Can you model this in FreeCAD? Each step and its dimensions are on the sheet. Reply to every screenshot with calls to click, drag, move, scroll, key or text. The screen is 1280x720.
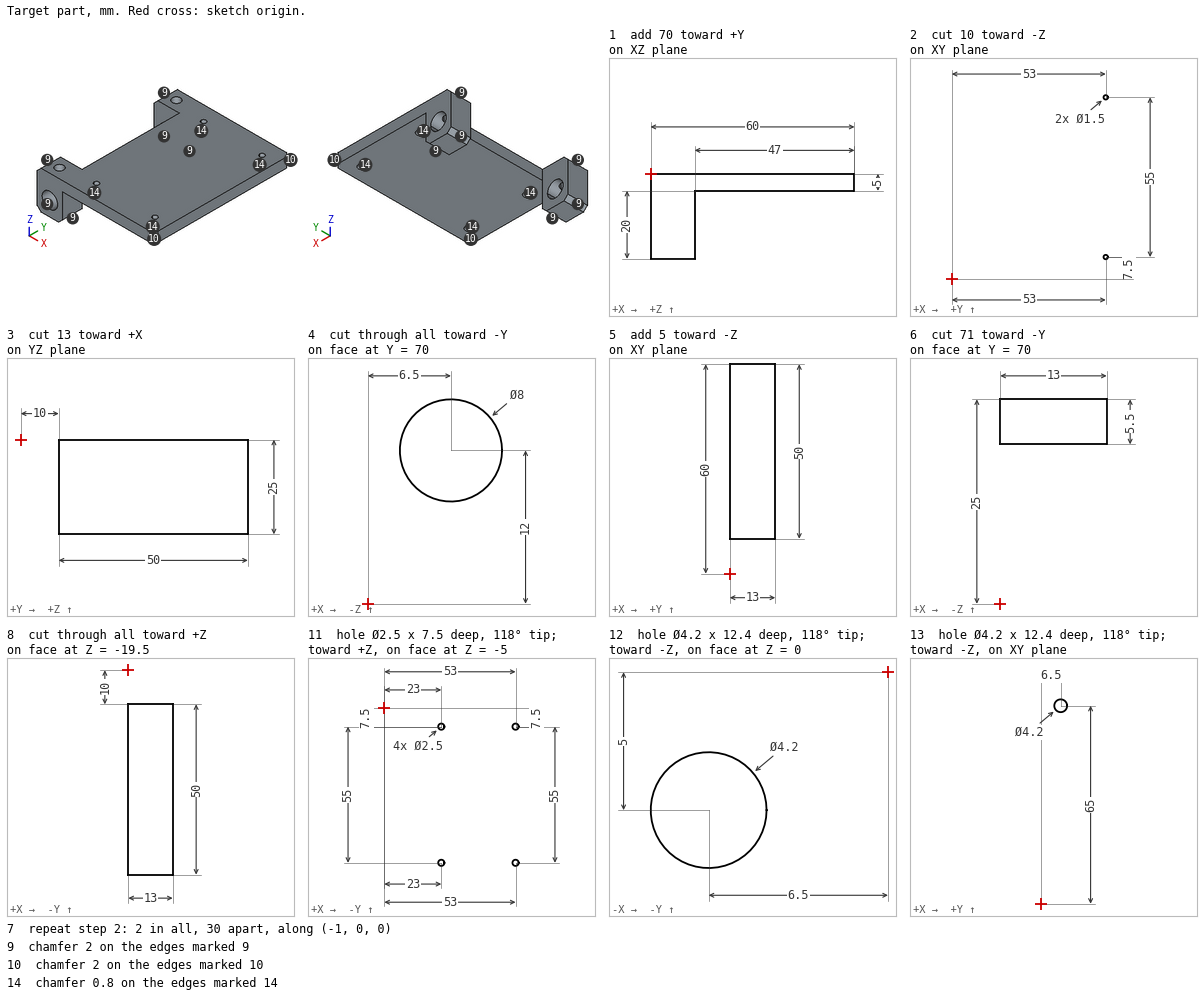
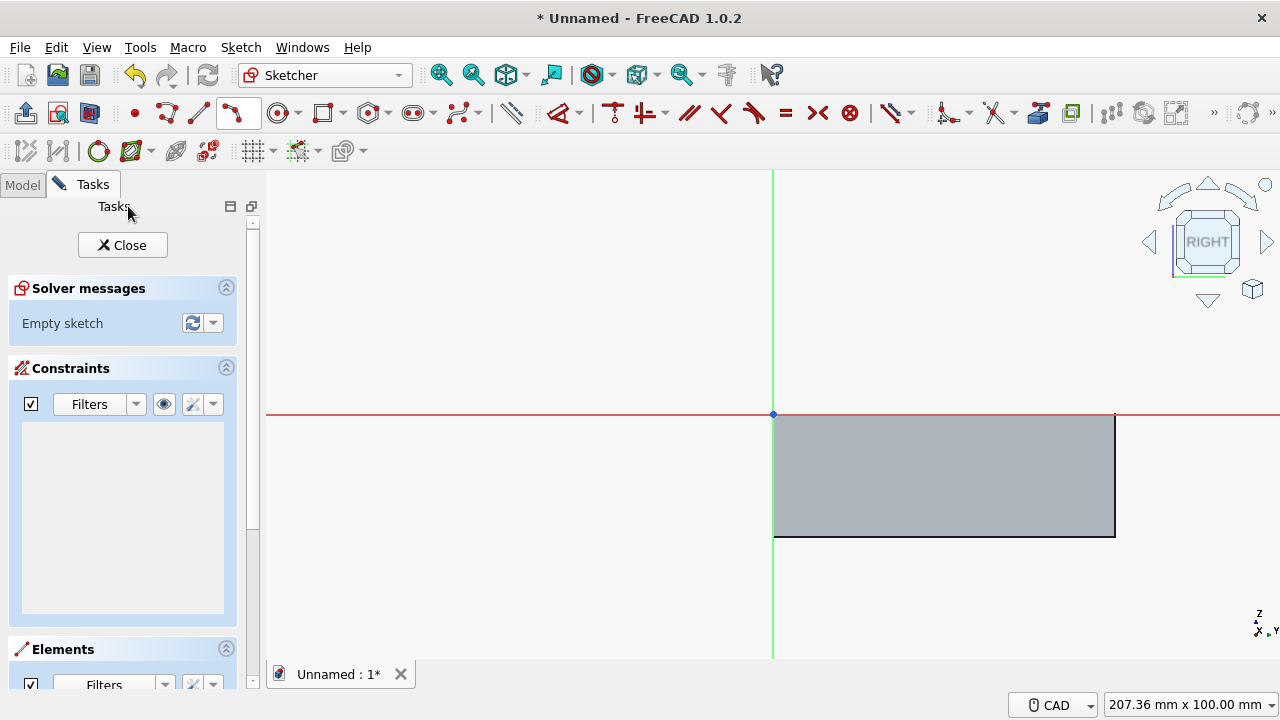
scroll(1115, 550, up, 3)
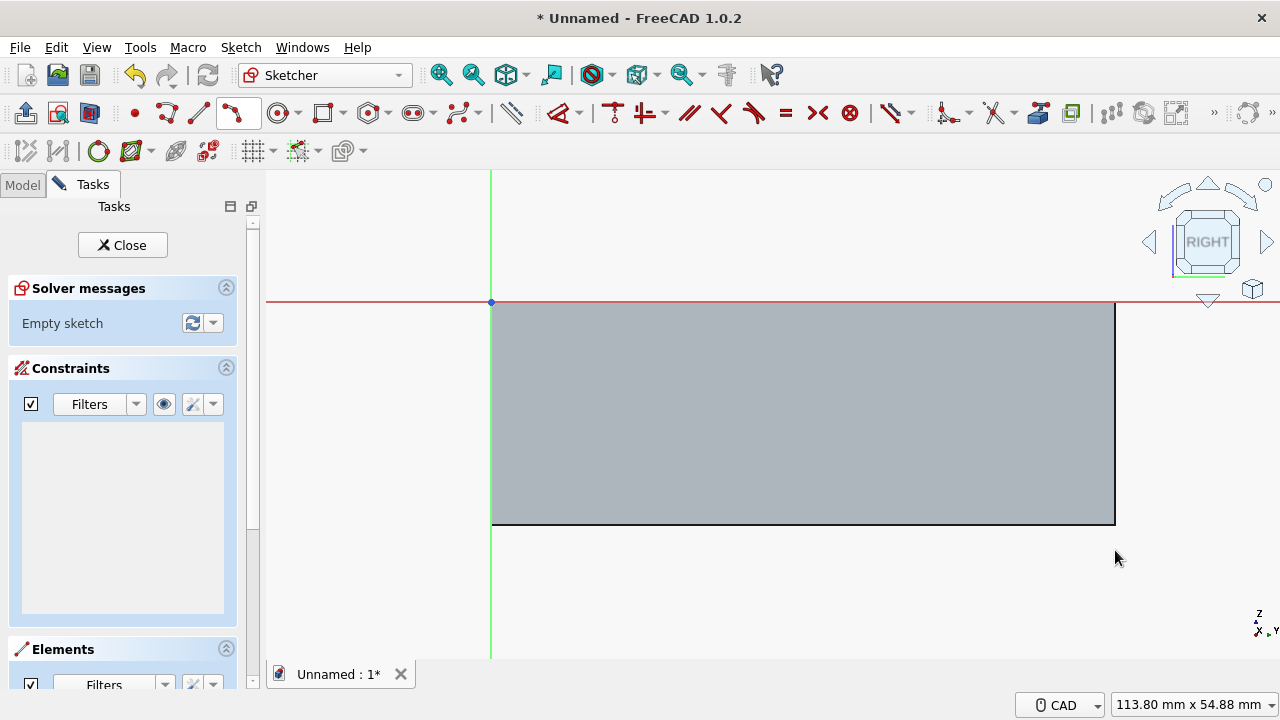
key(g)
key(r)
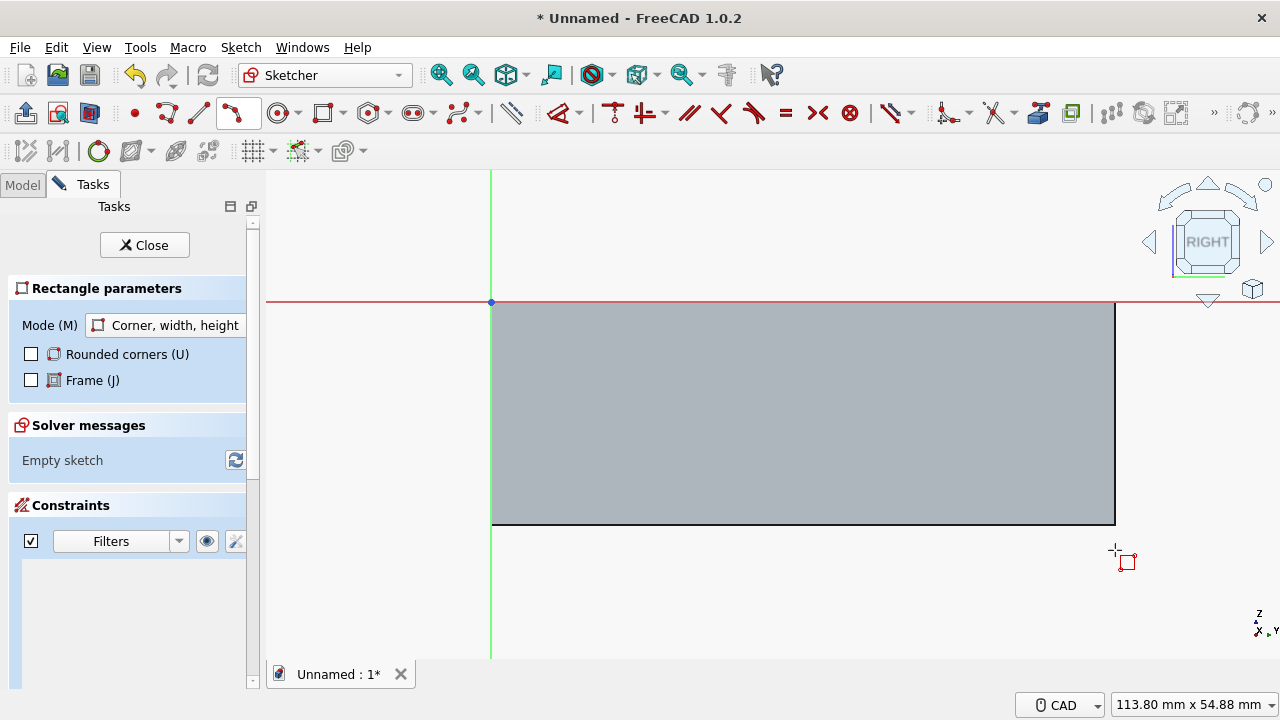
click(580, 302)
move(1026, 525)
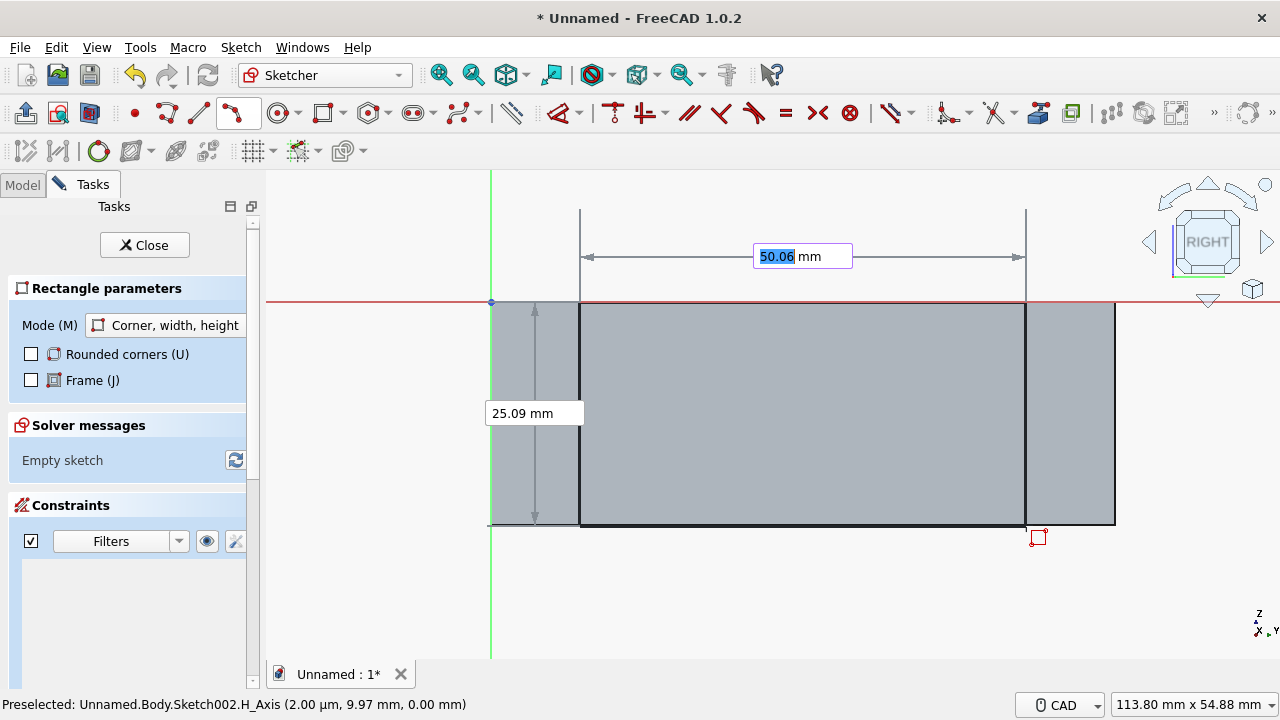
text(50)
key(Tab)
text(25)
key(Return)
key(Escape)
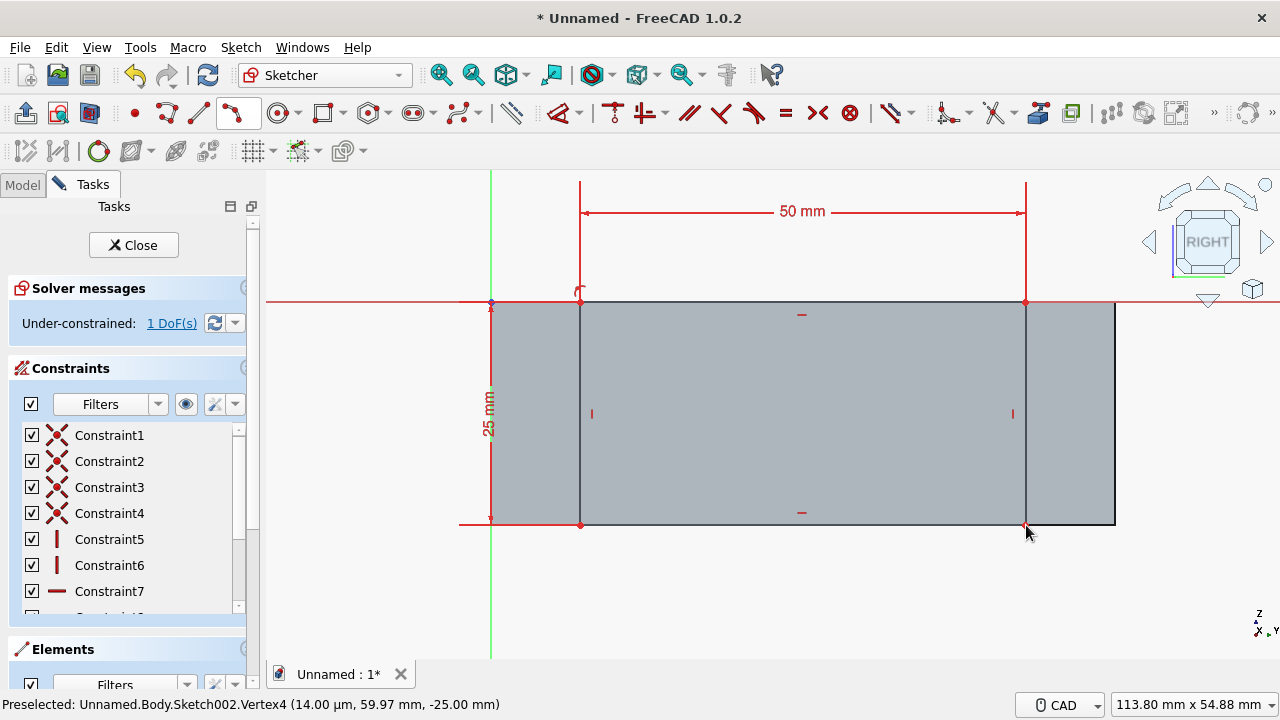
key(d)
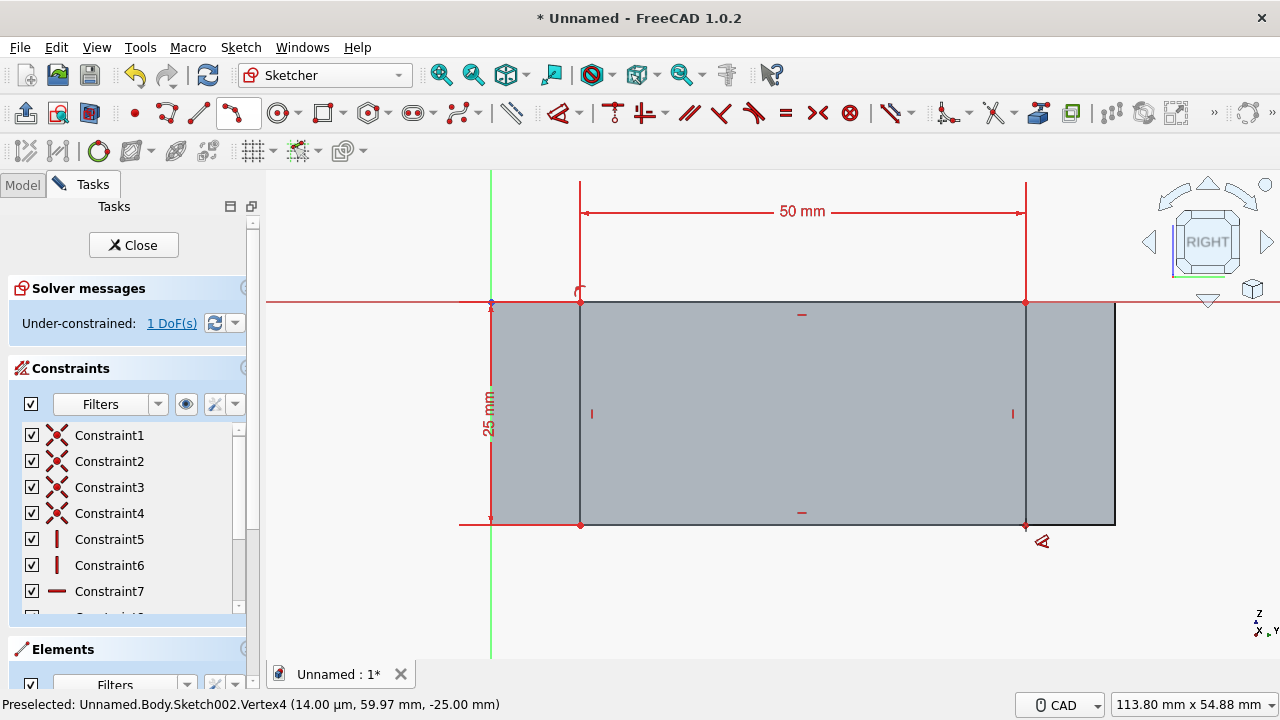
click(580, 302)
click(536, 268)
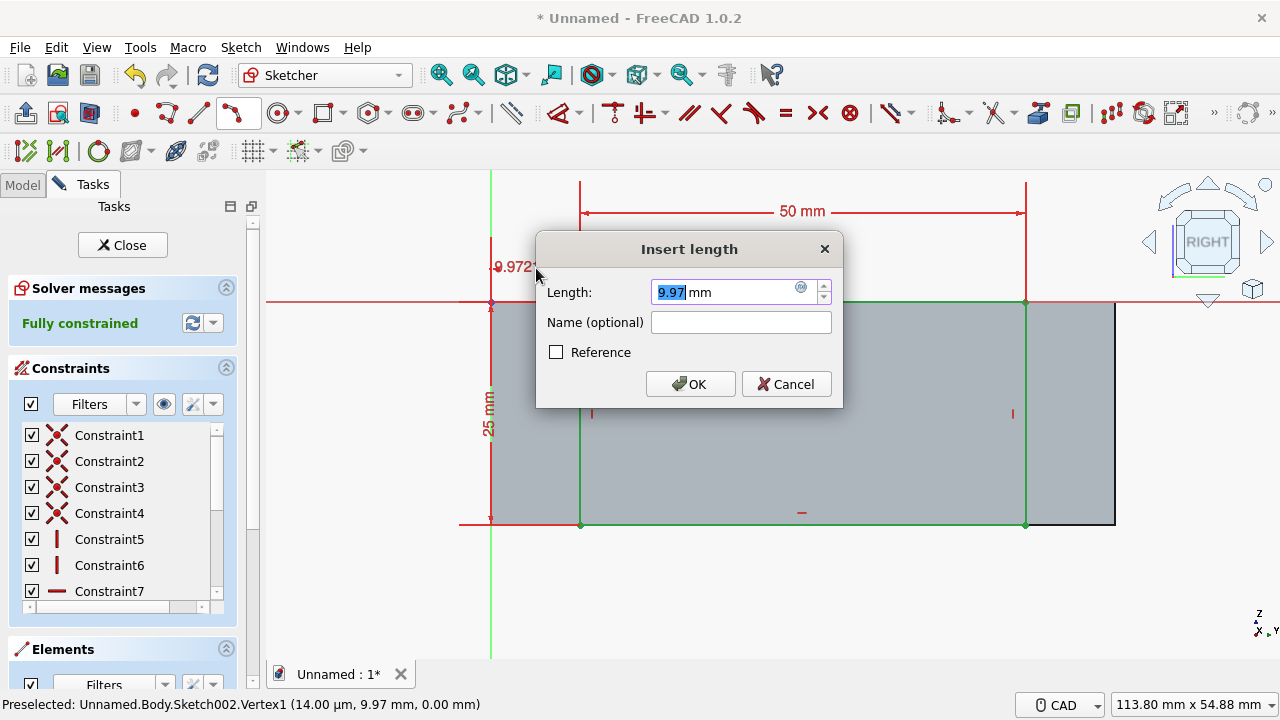
text(10)
key(Return)
key(Escape)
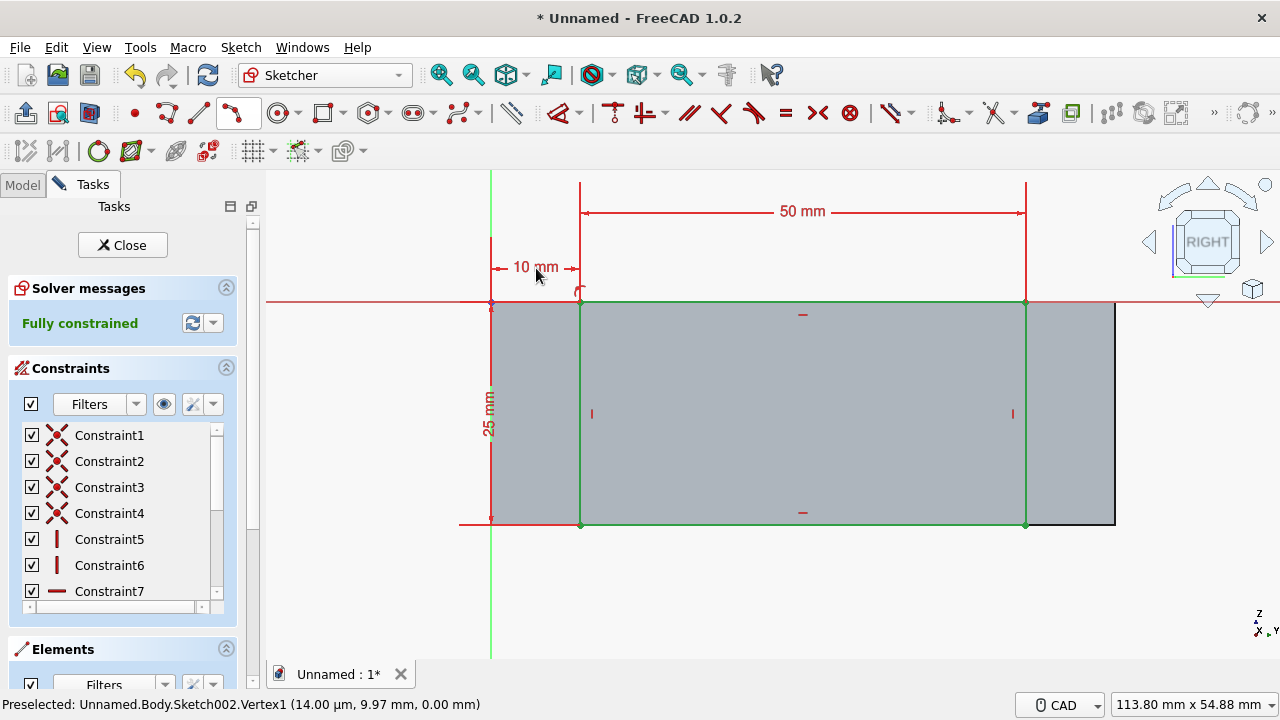
click(123, 245)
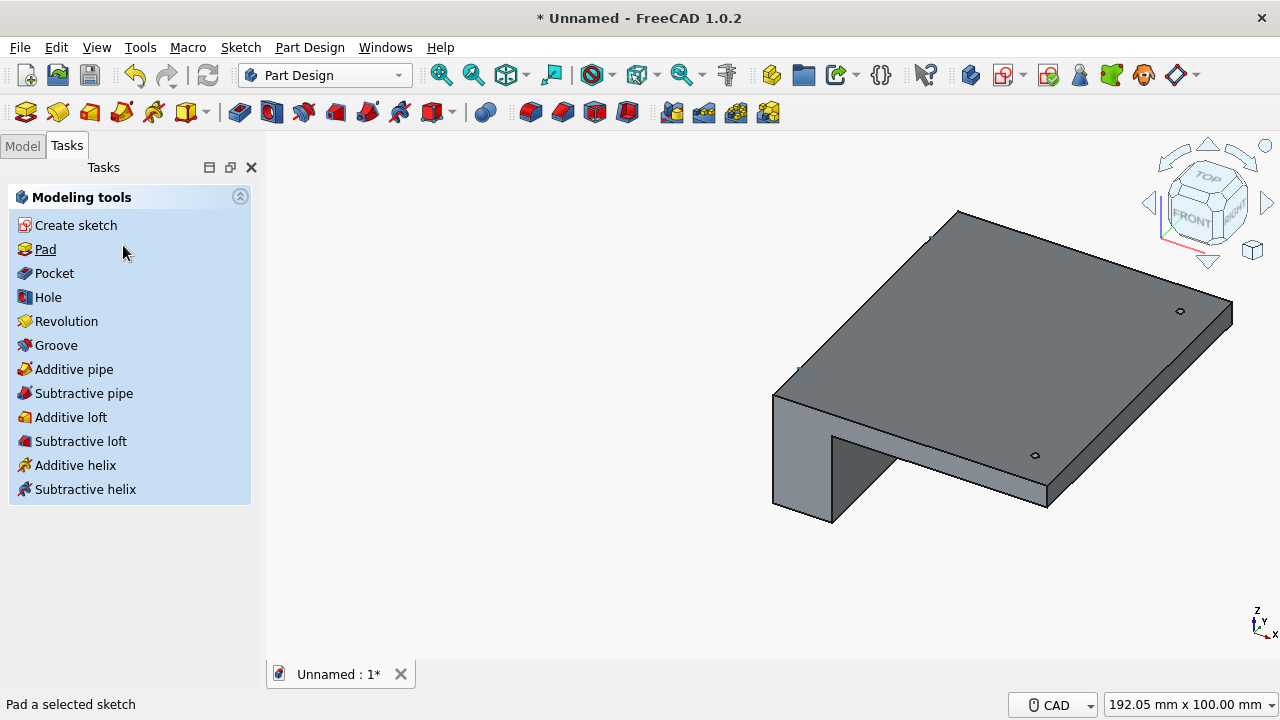
click(240, 112)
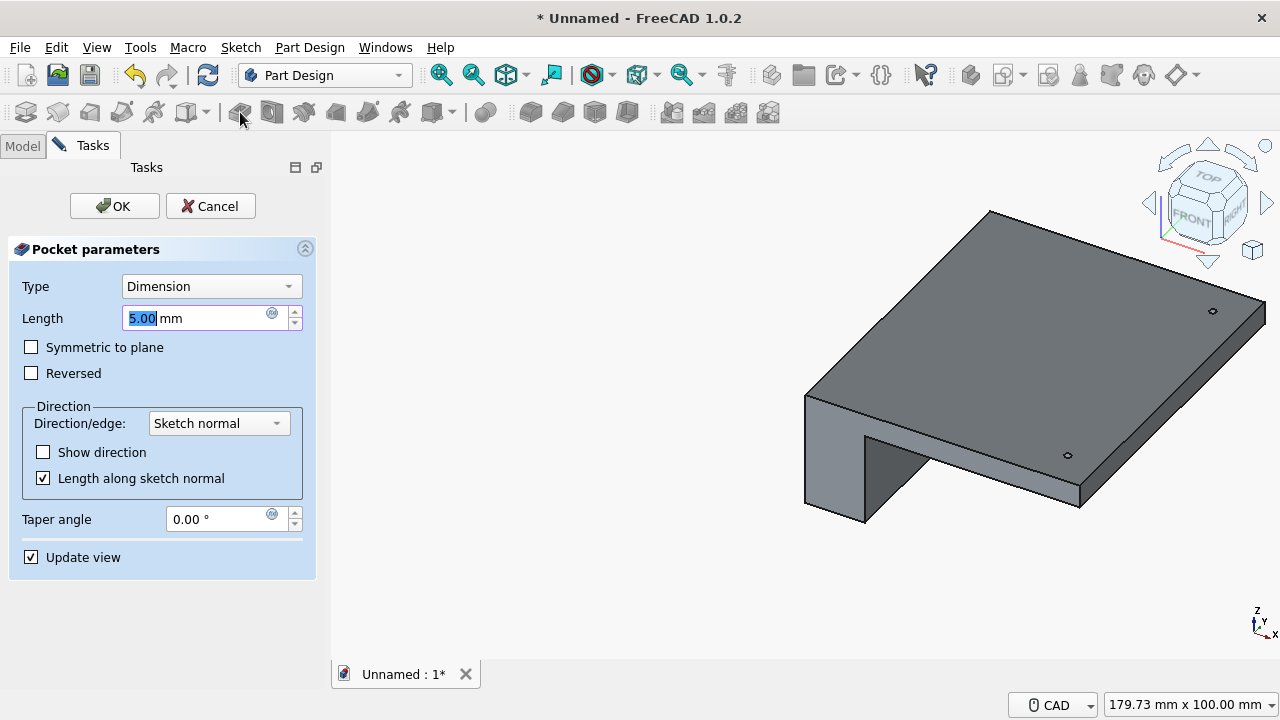
text(13)
key(Tab)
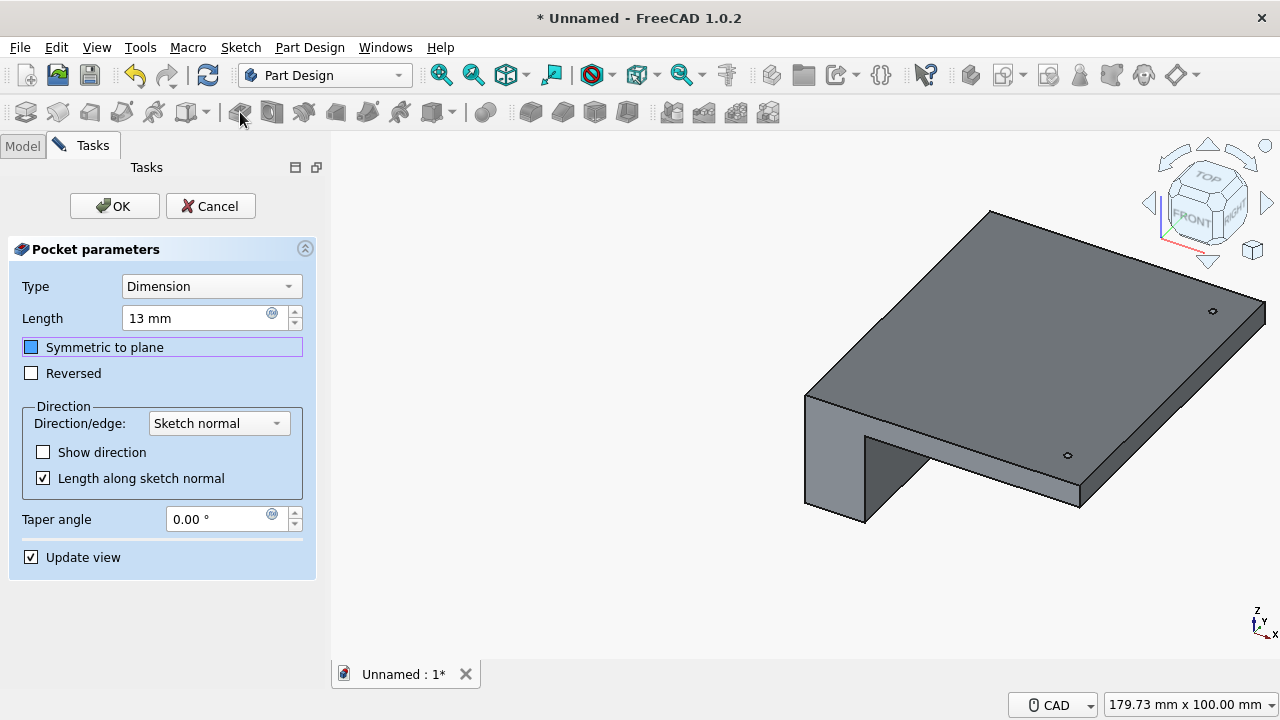
click(30, 373)